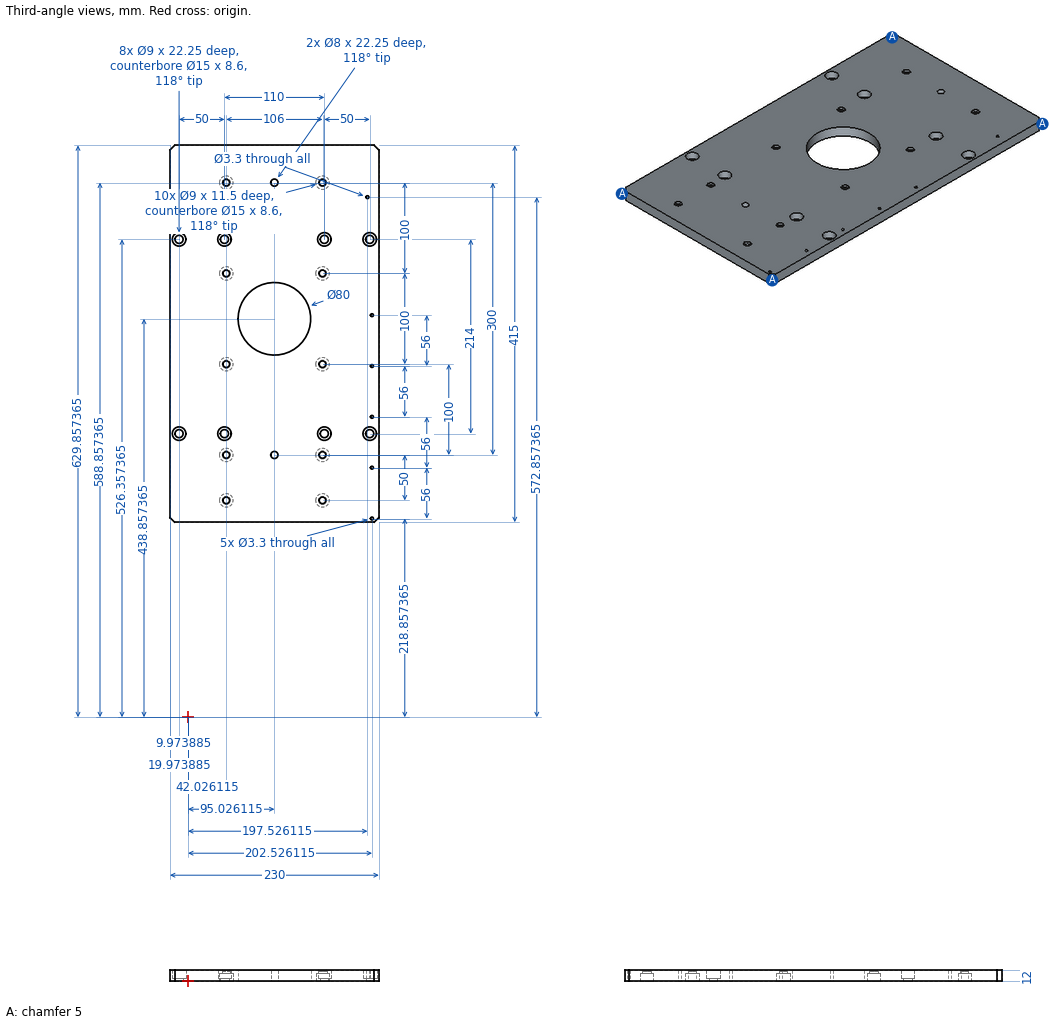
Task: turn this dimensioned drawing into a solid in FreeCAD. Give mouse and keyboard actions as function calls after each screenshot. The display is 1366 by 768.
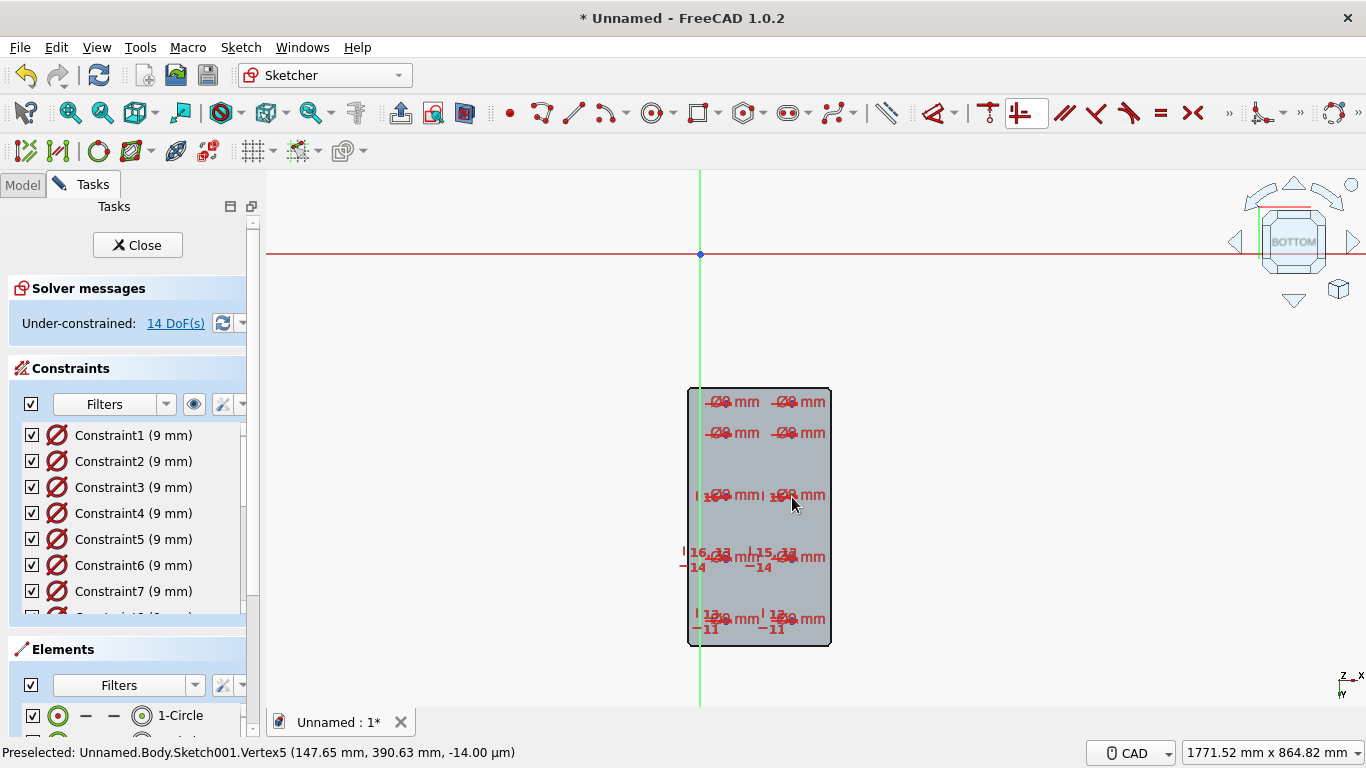
click(726, 497)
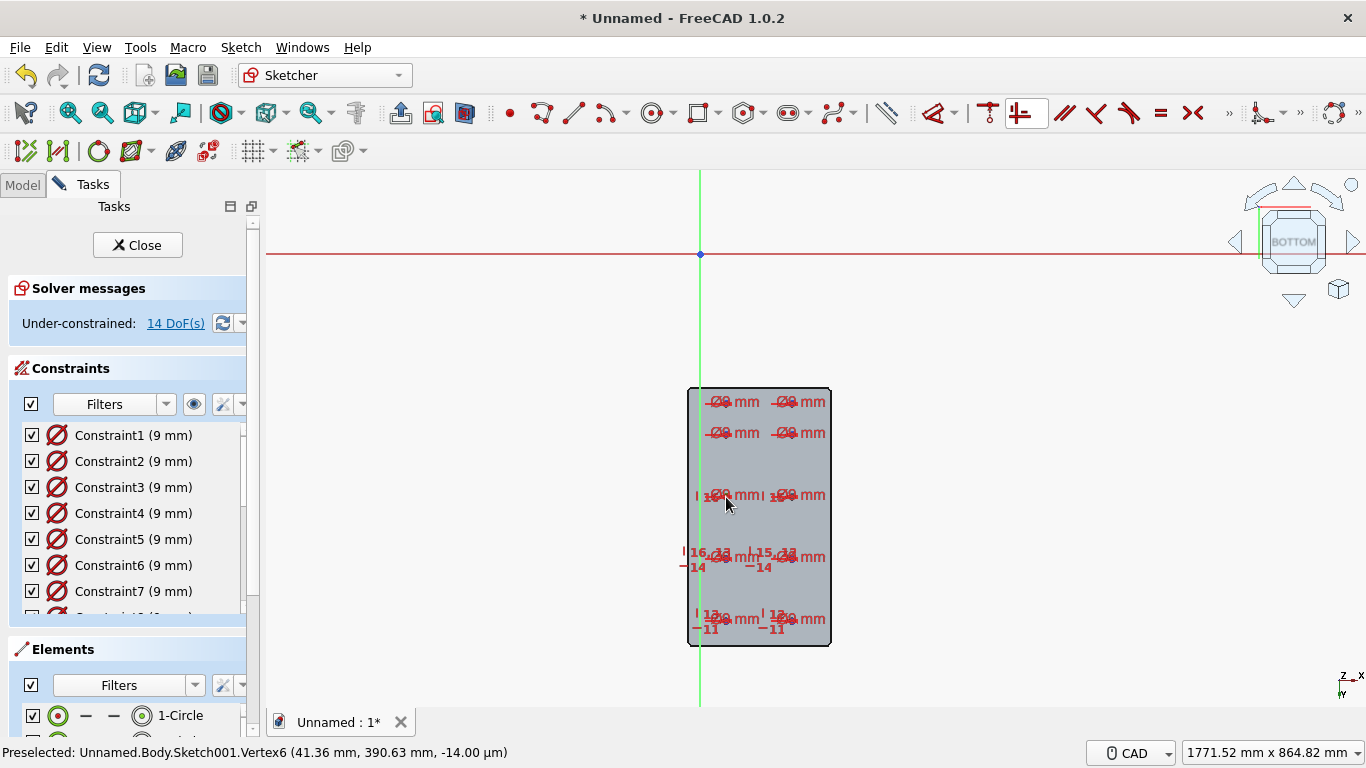
click(1042, 114)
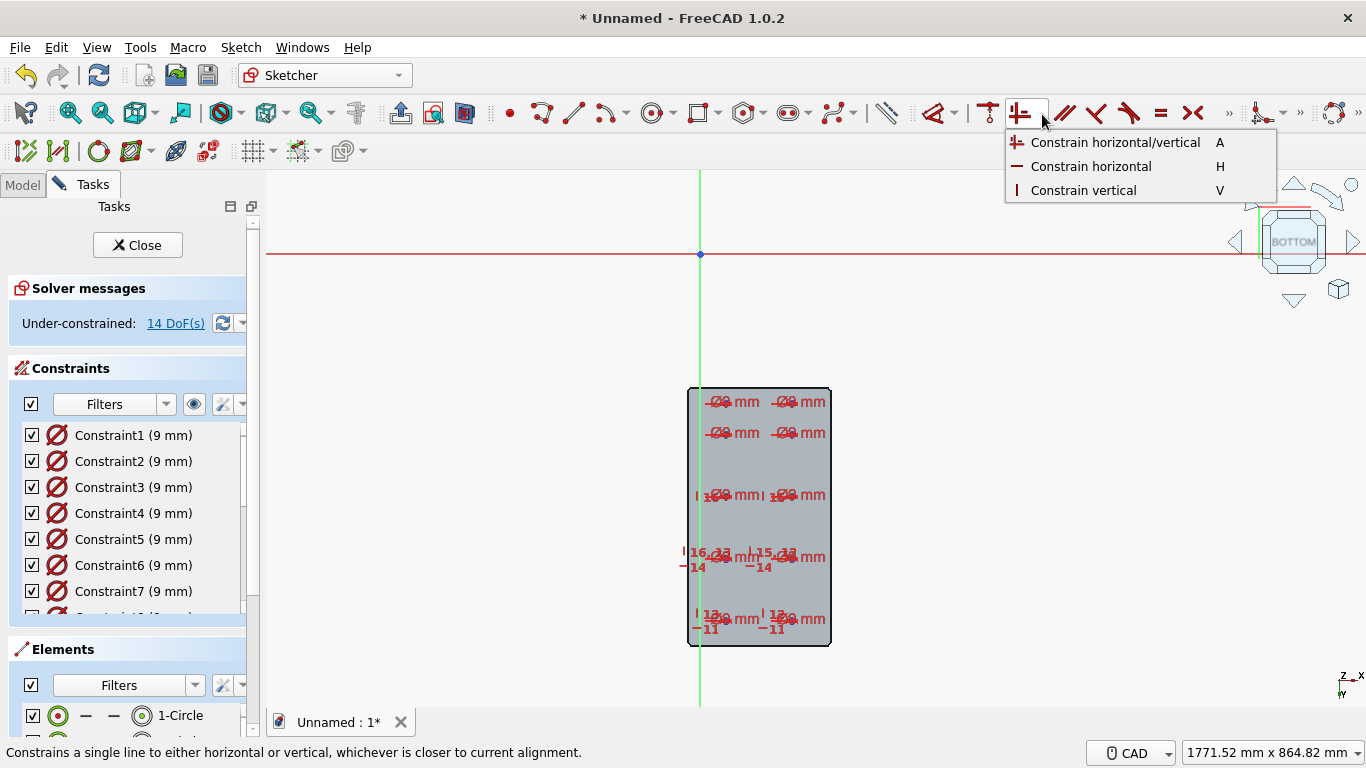
click(1141, 166)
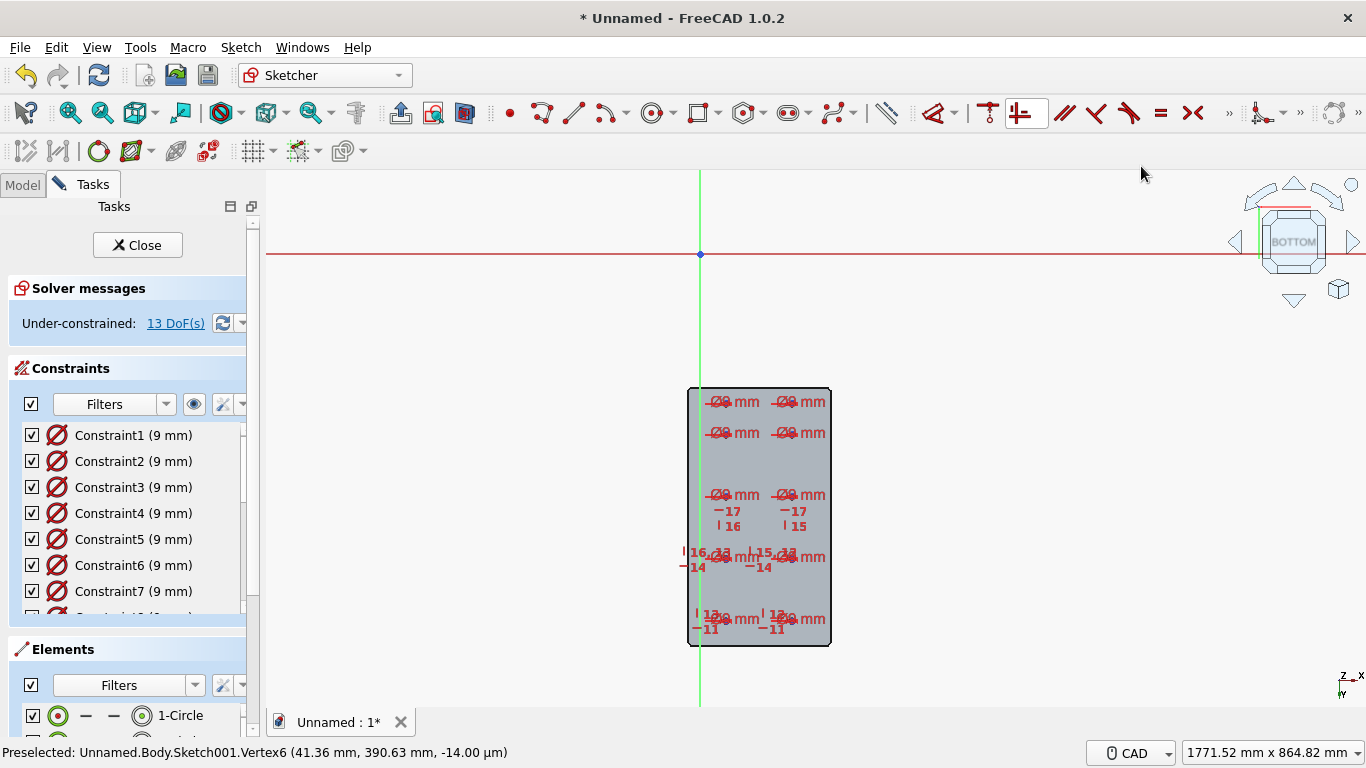
click(792, 497)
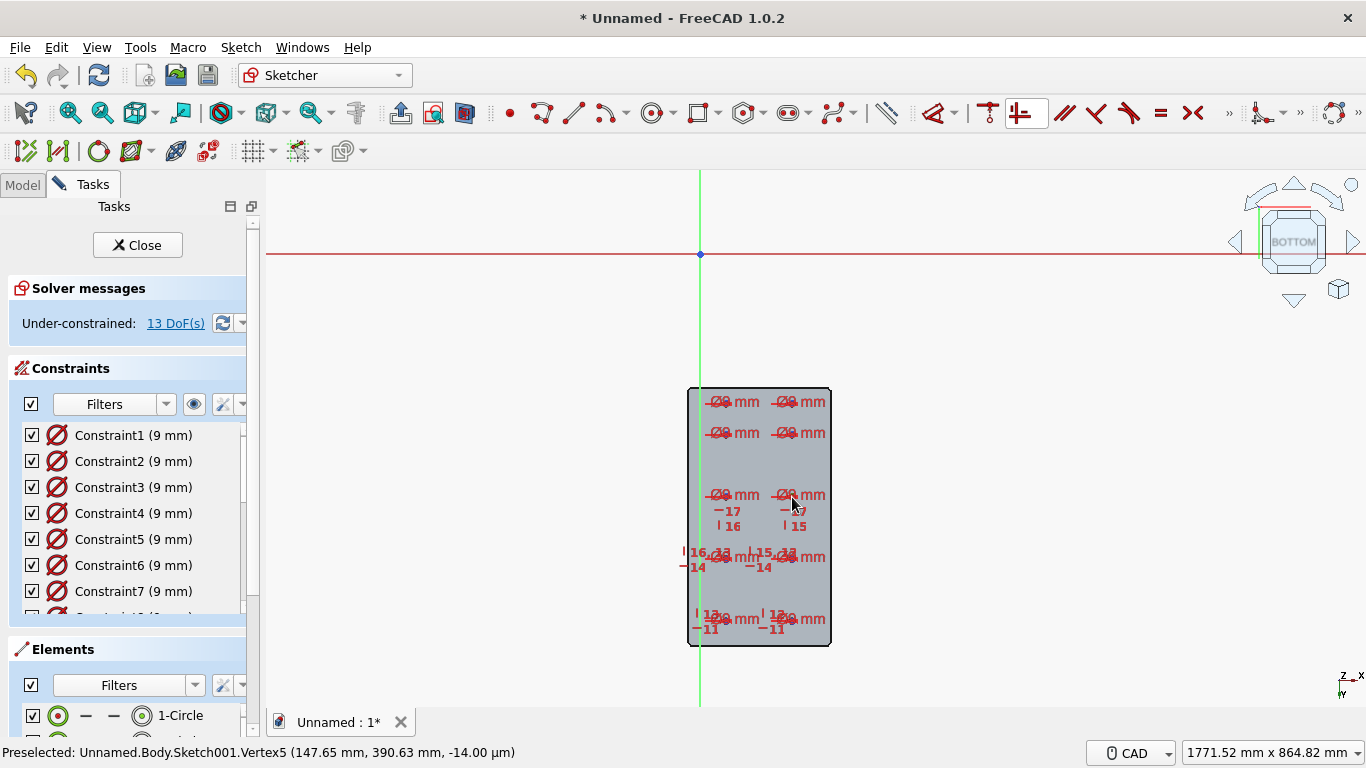
click(792, 435)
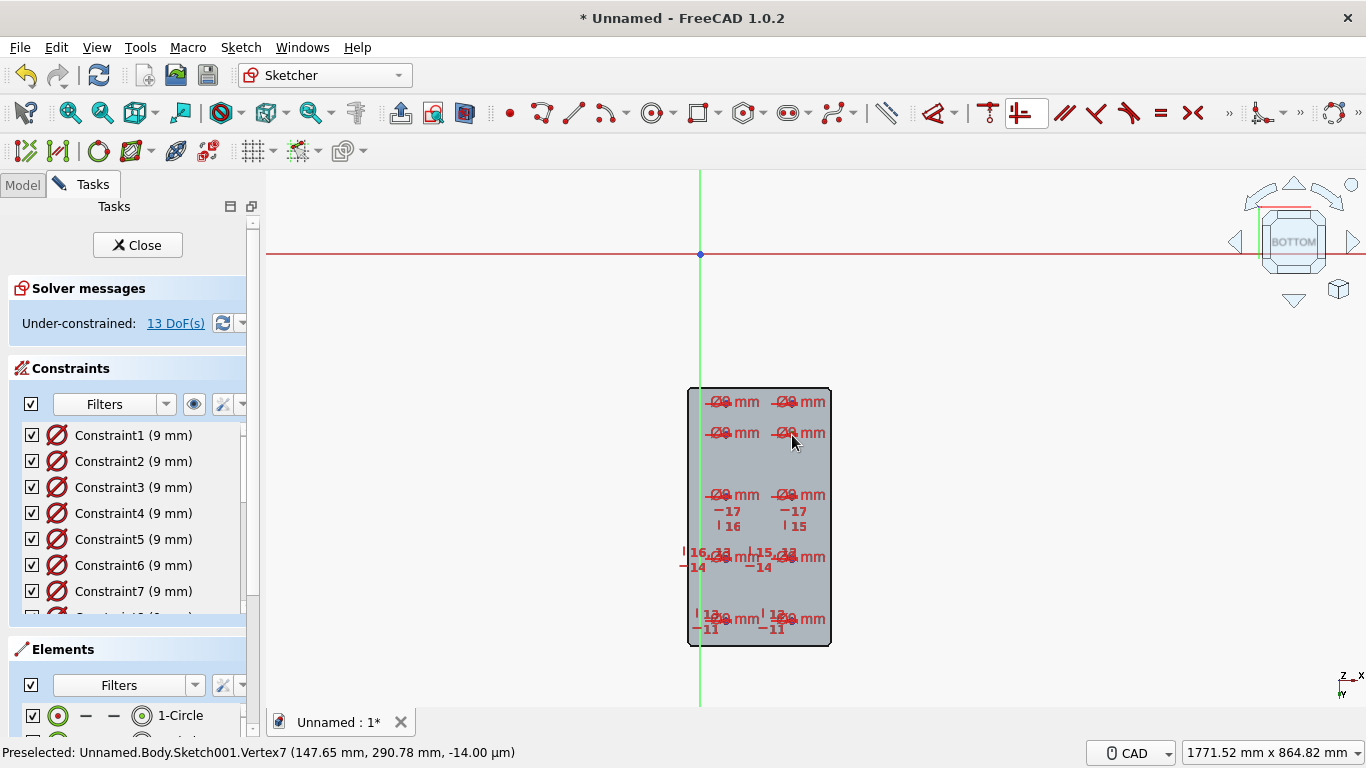
key(v)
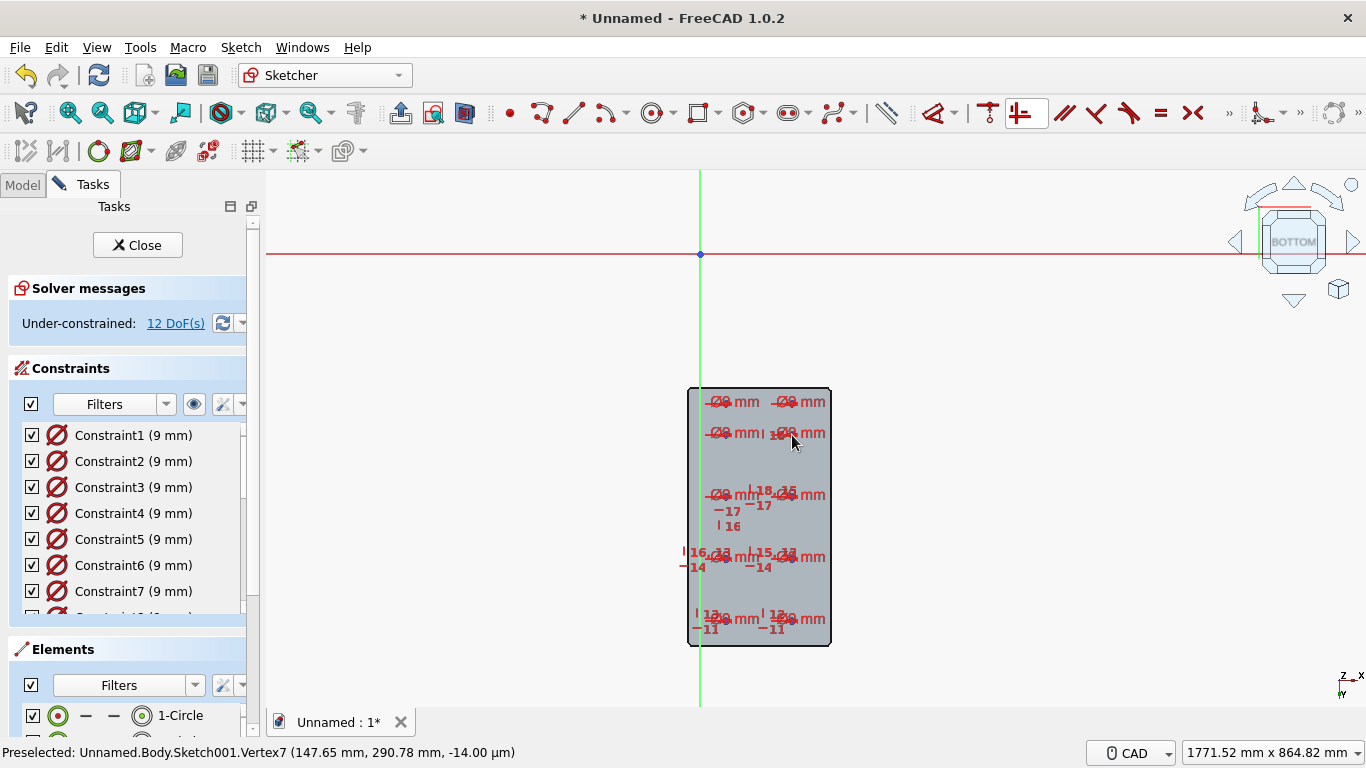
click(726, 497)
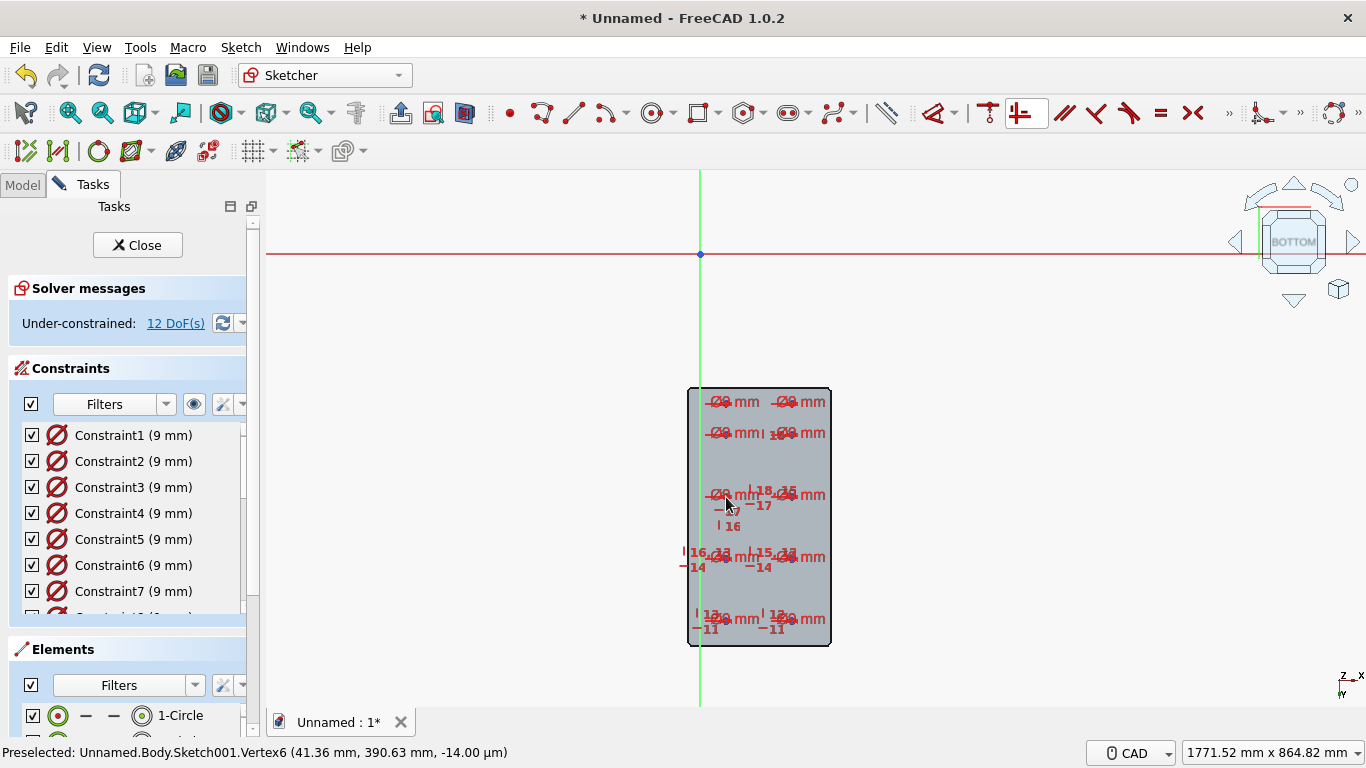
click(726, 435)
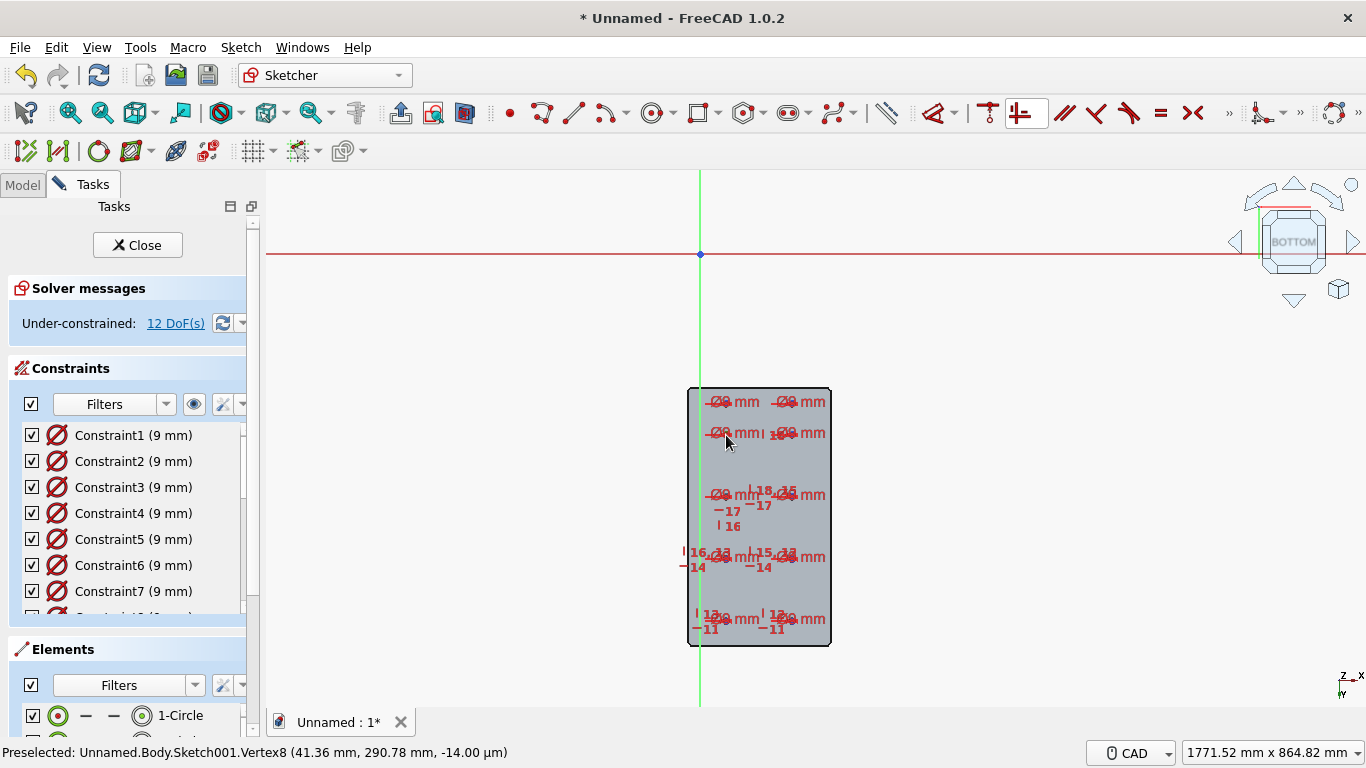
key(v)